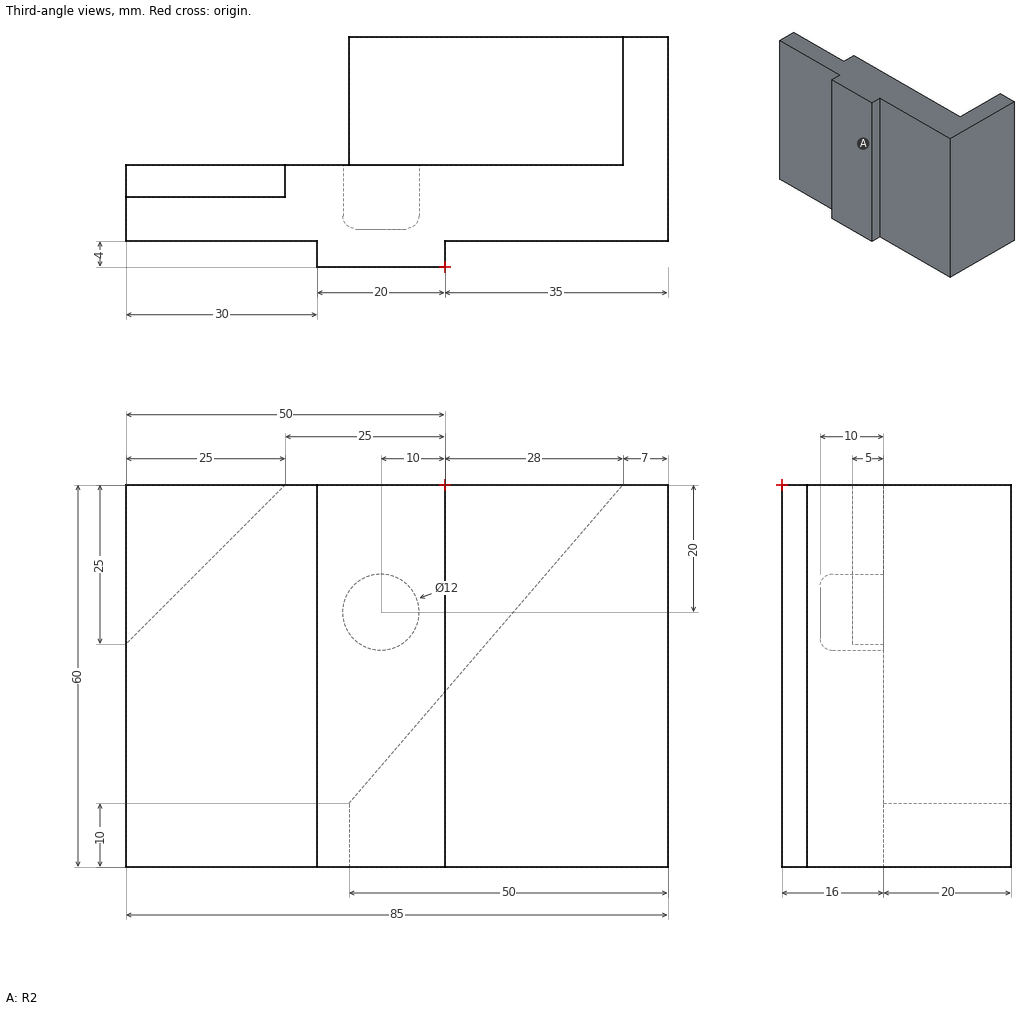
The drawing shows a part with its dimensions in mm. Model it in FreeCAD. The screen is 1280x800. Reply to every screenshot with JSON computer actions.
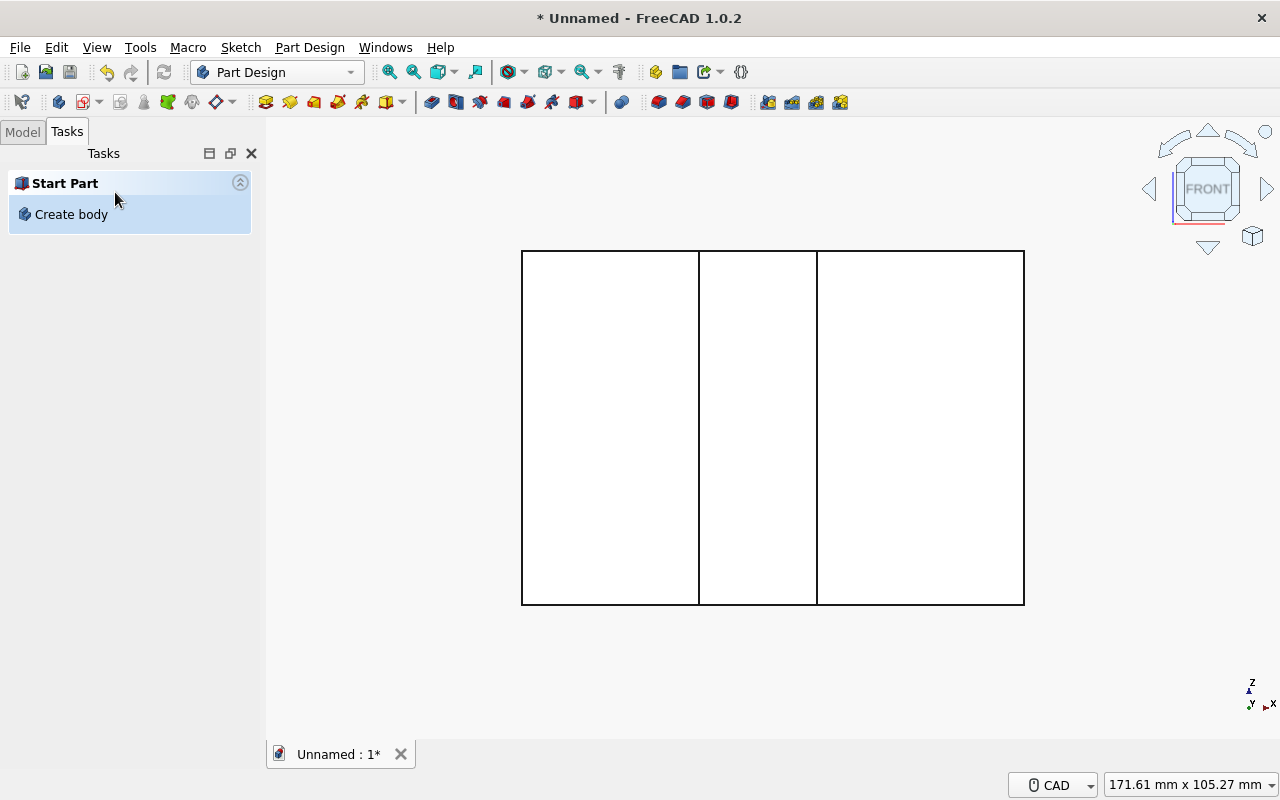
{"action": "key", "text": "3"}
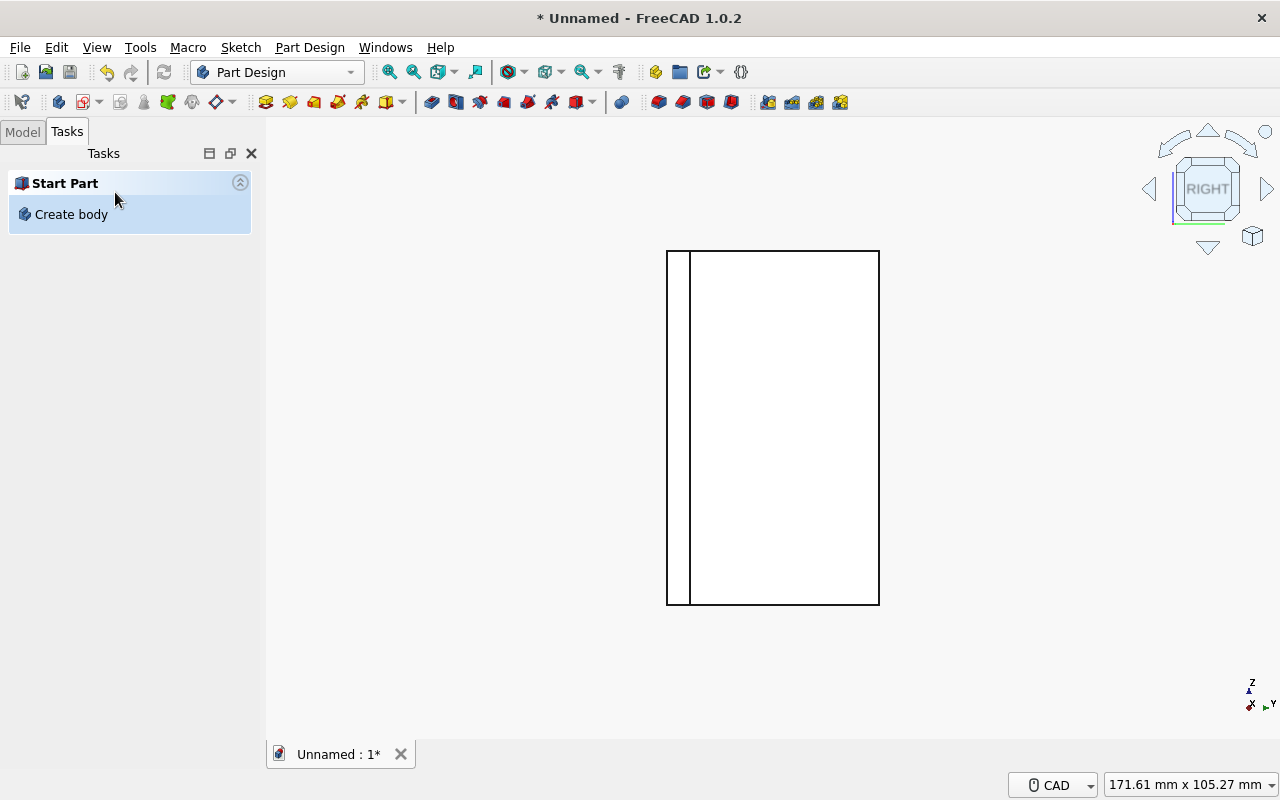
{"action": "key", "text": "5"}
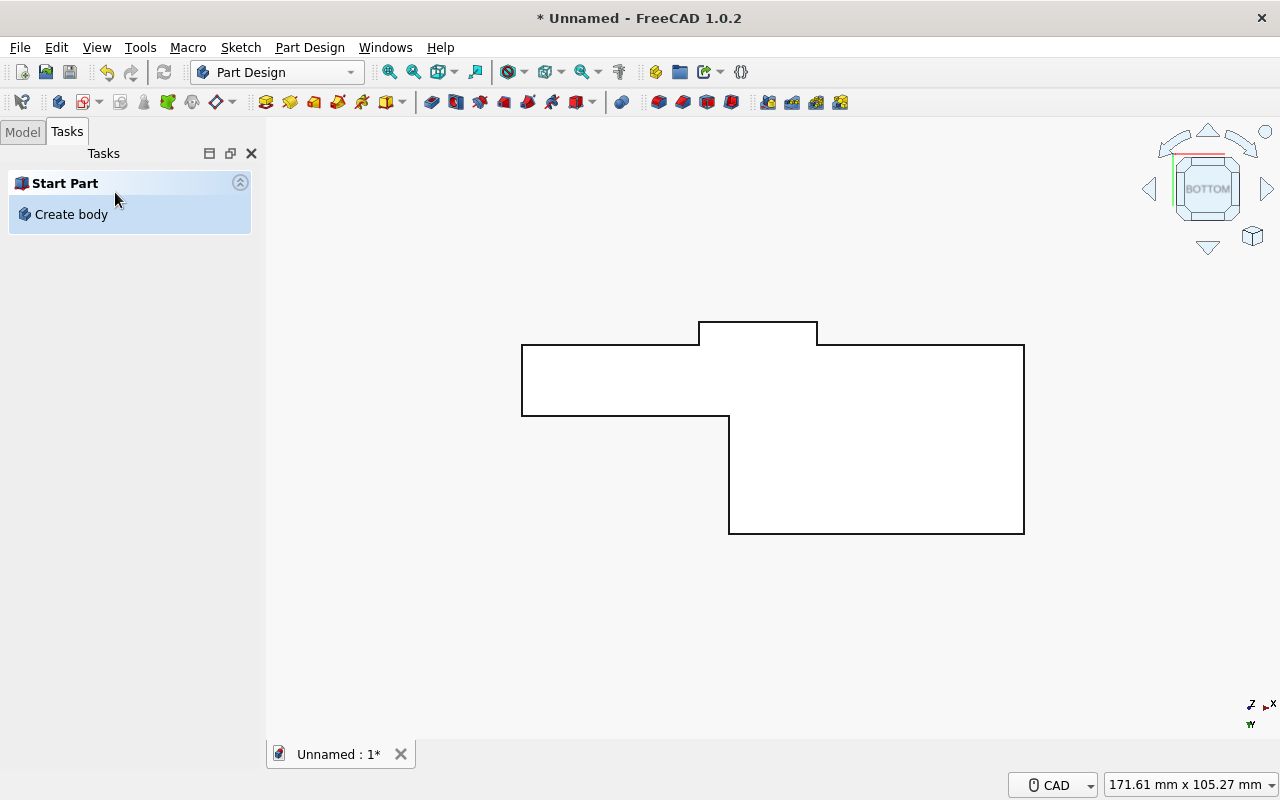
{"action": "key", "text": "4"}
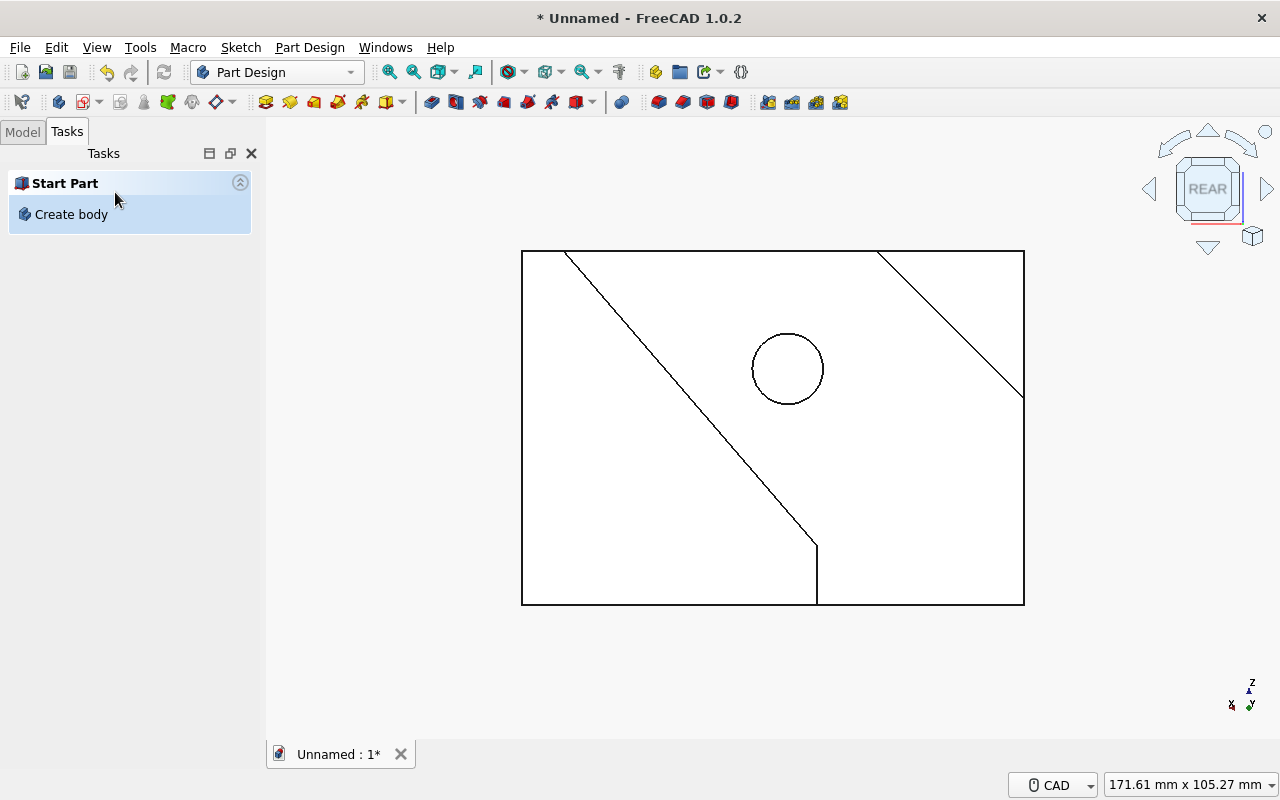
{"action": "key", "text": "6"}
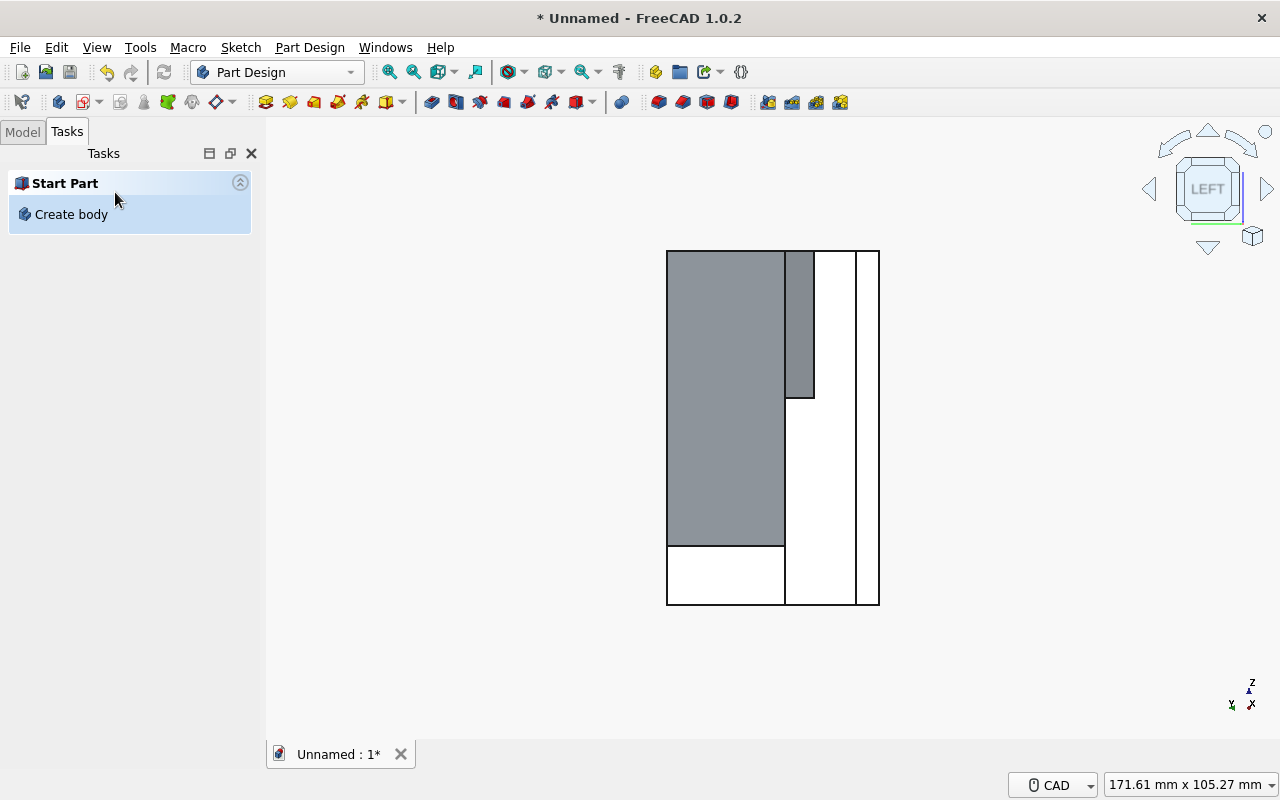
{"action": "key", "text": "v 3"}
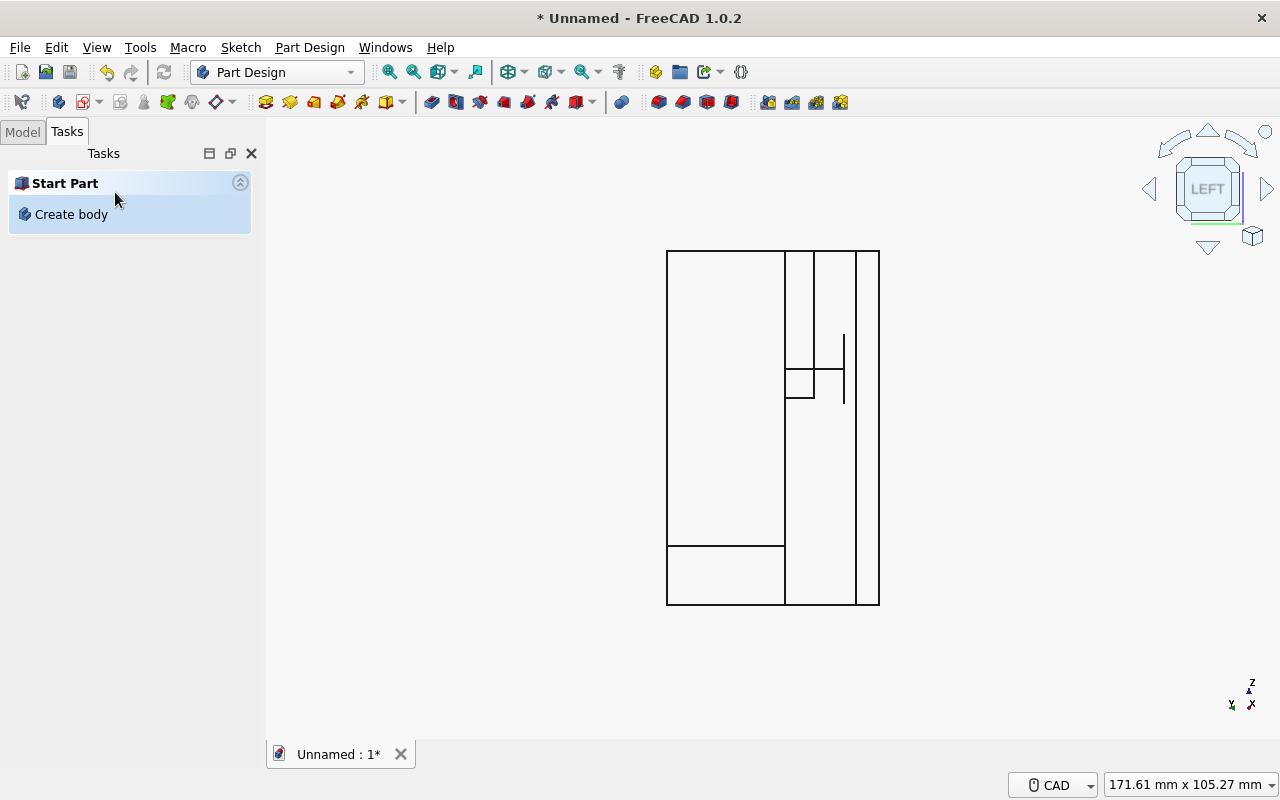
{"action": "key", "text": "0"}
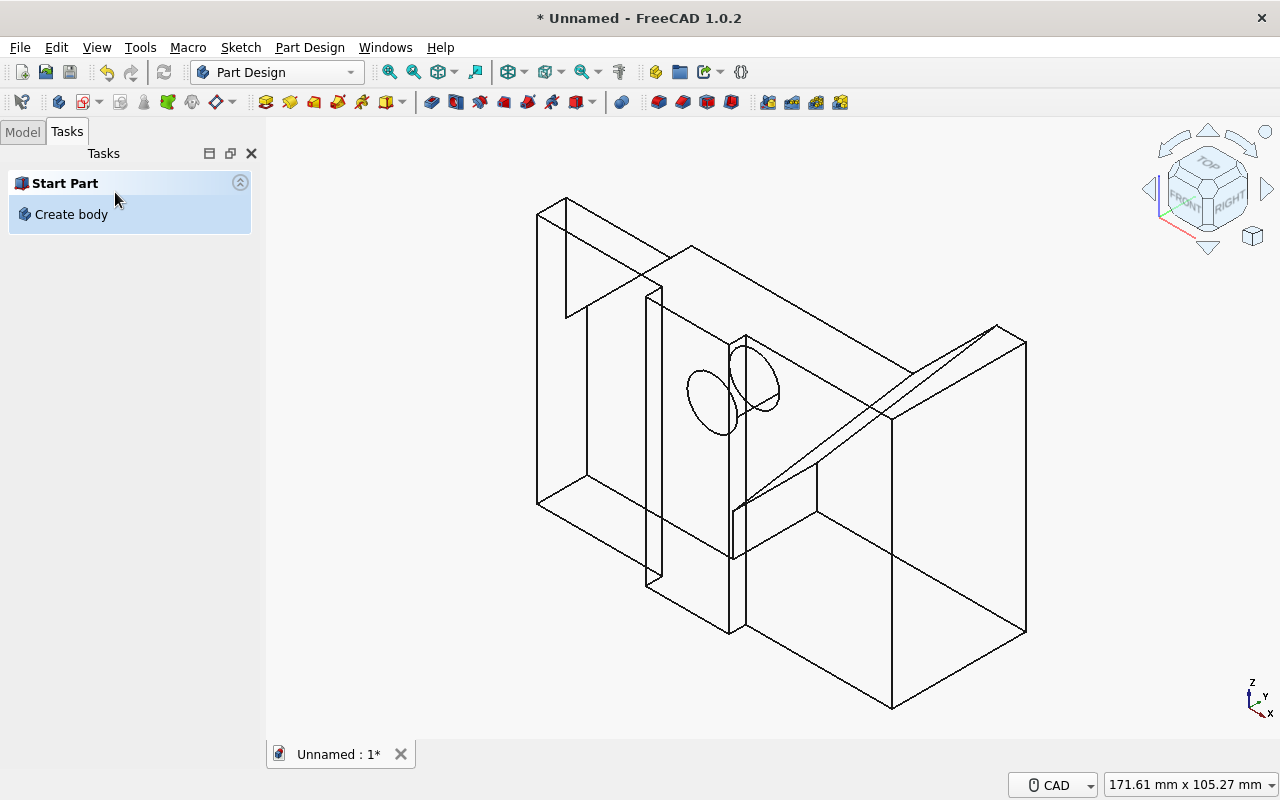
{"action": "left_click", "coordinate": [687, 387]}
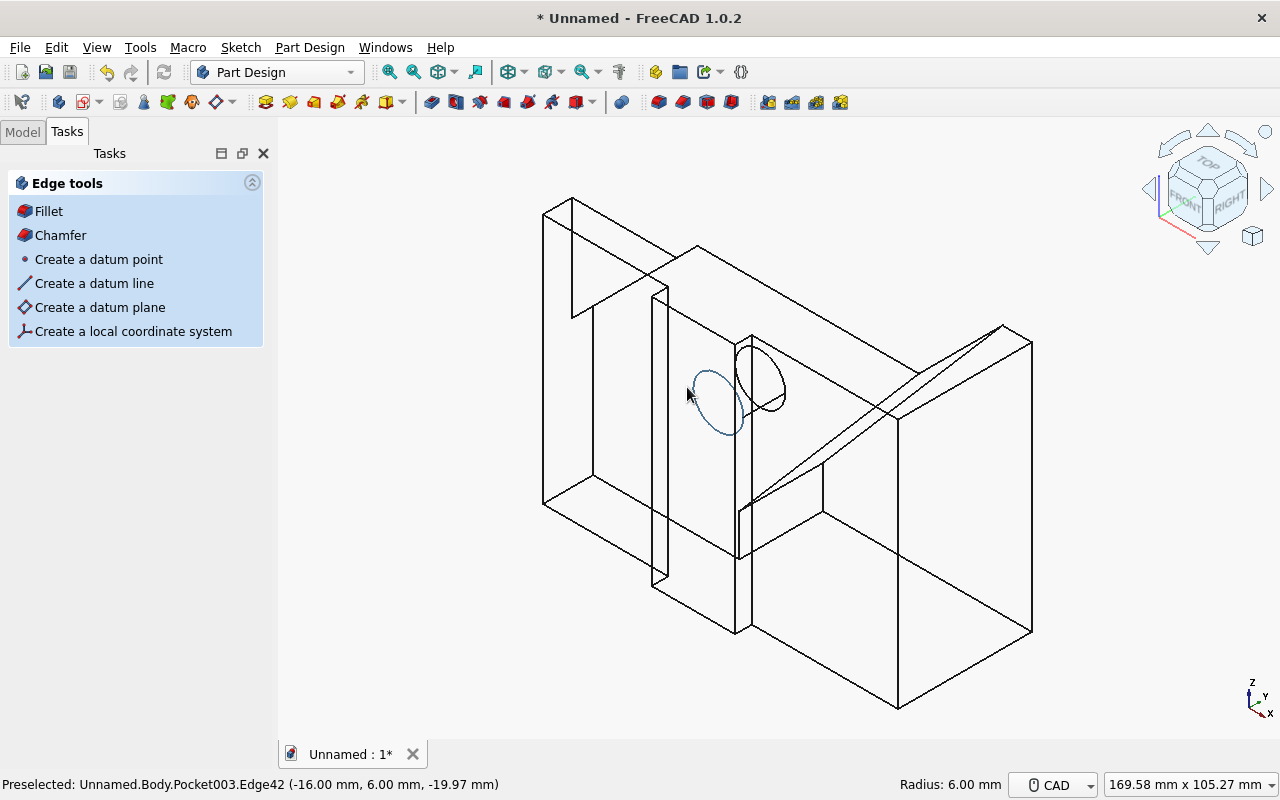
{"action": "key", "text": "v 1"}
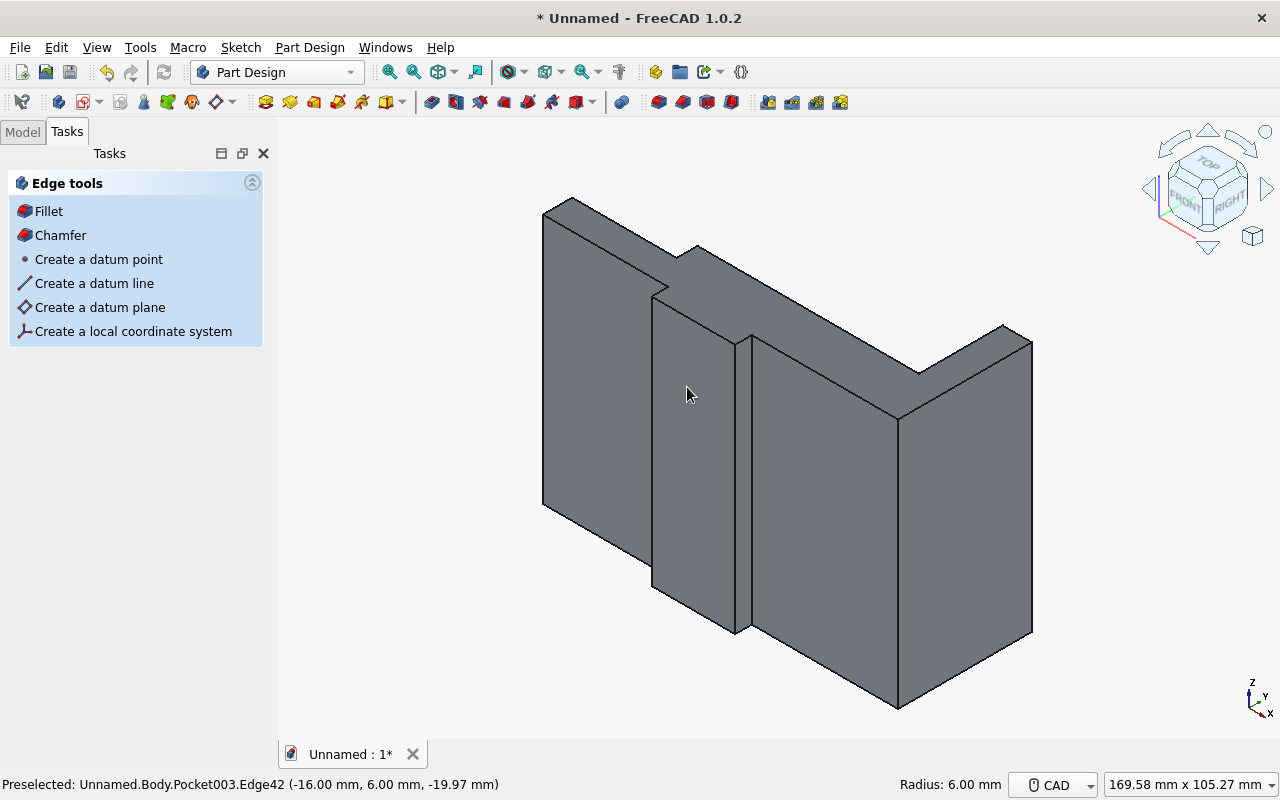
{"action": "left_click", "coordinate": [660, 102]}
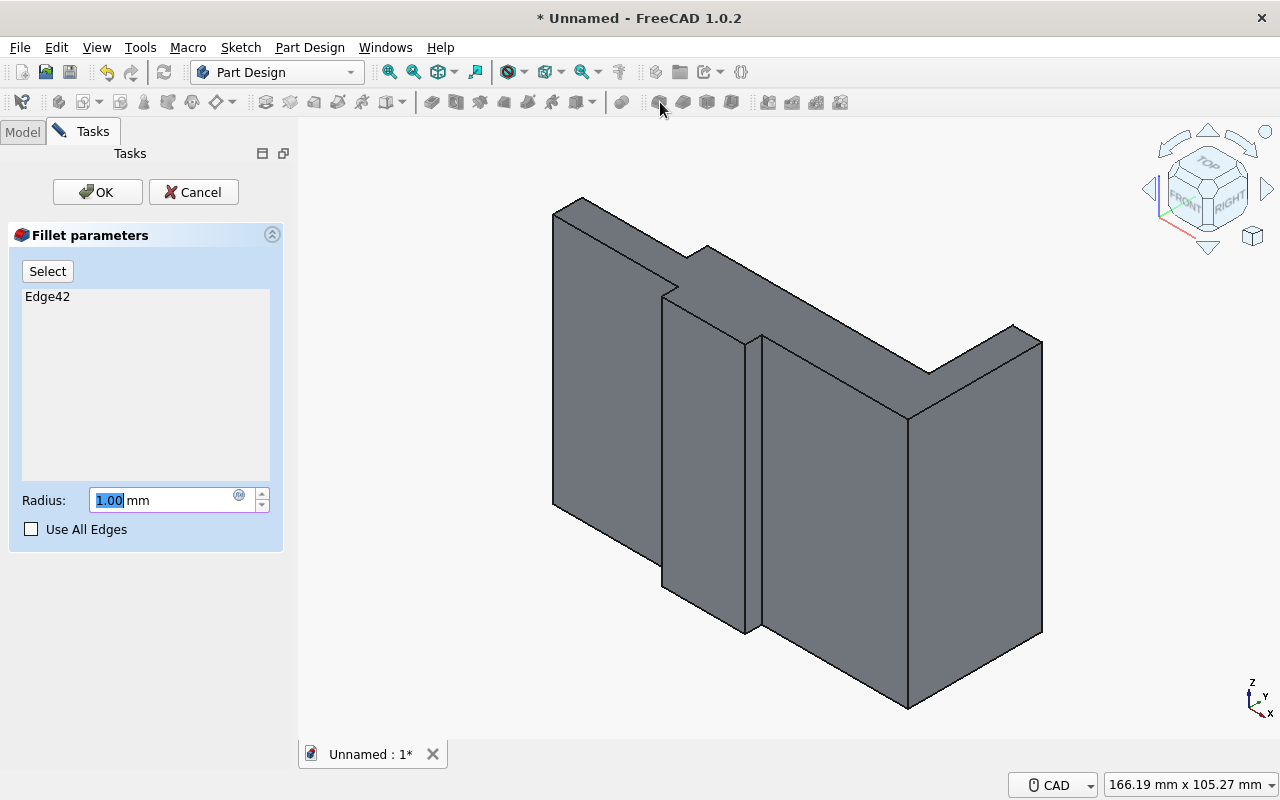
{"action": "type", "text": "2"}
{"action": "key", "text": "Tab"}